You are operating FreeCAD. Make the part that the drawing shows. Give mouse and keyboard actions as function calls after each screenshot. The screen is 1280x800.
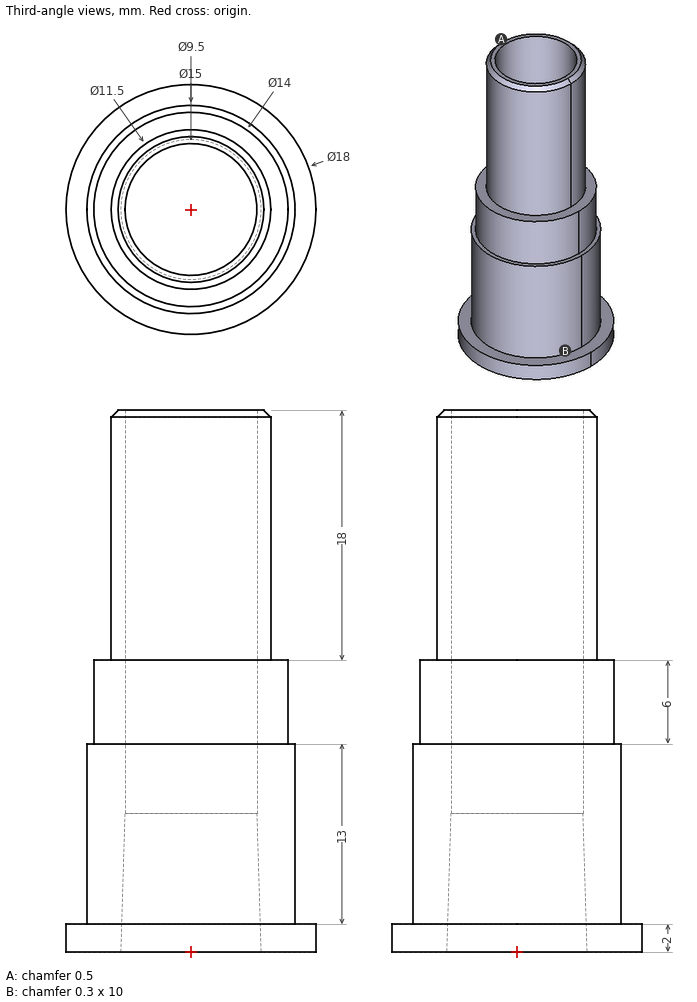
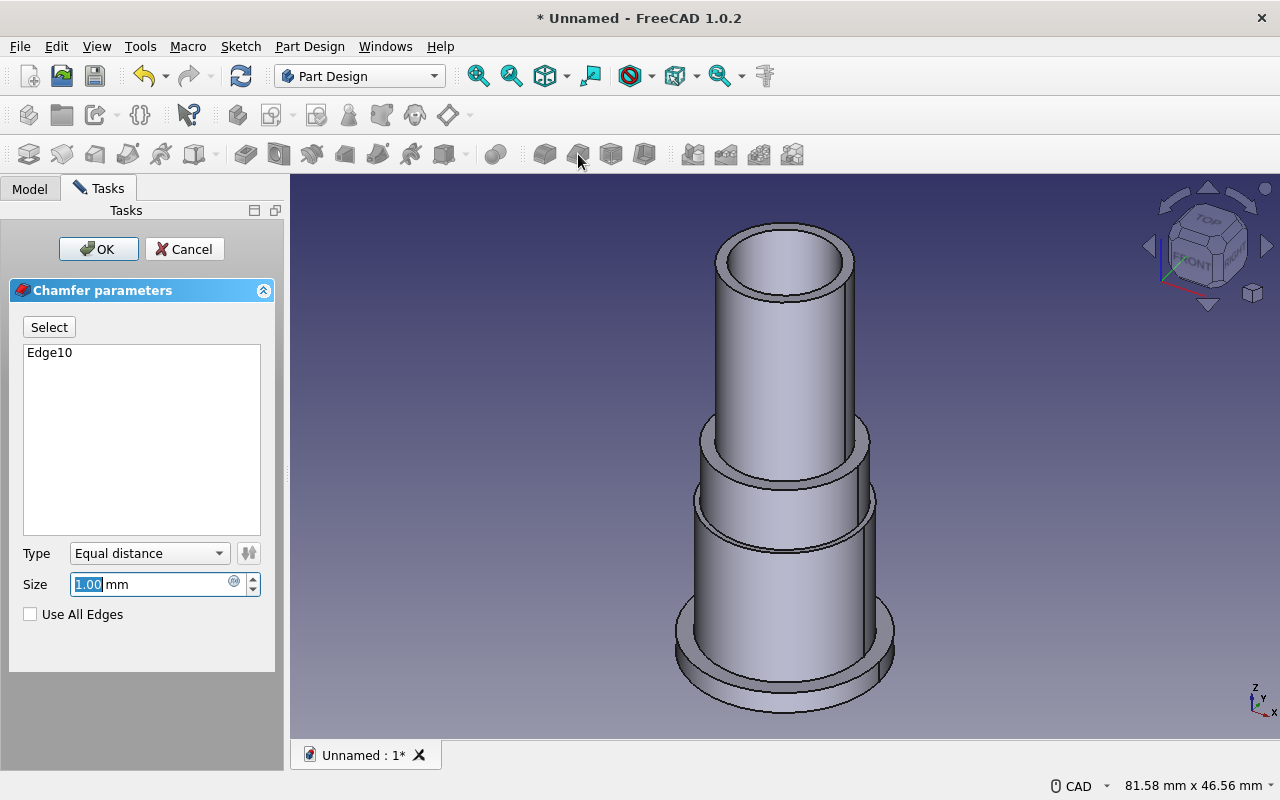
text(0.5)
key(Tab)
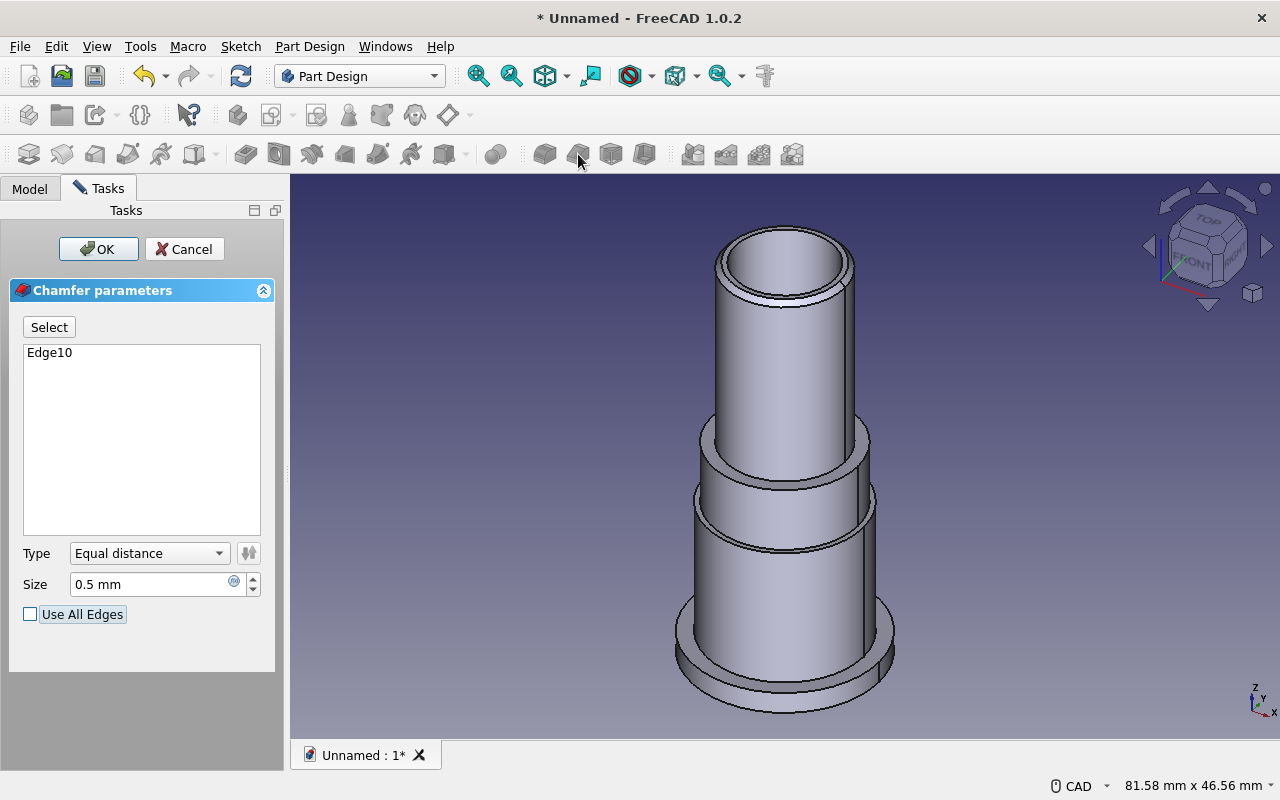
click(99, 249)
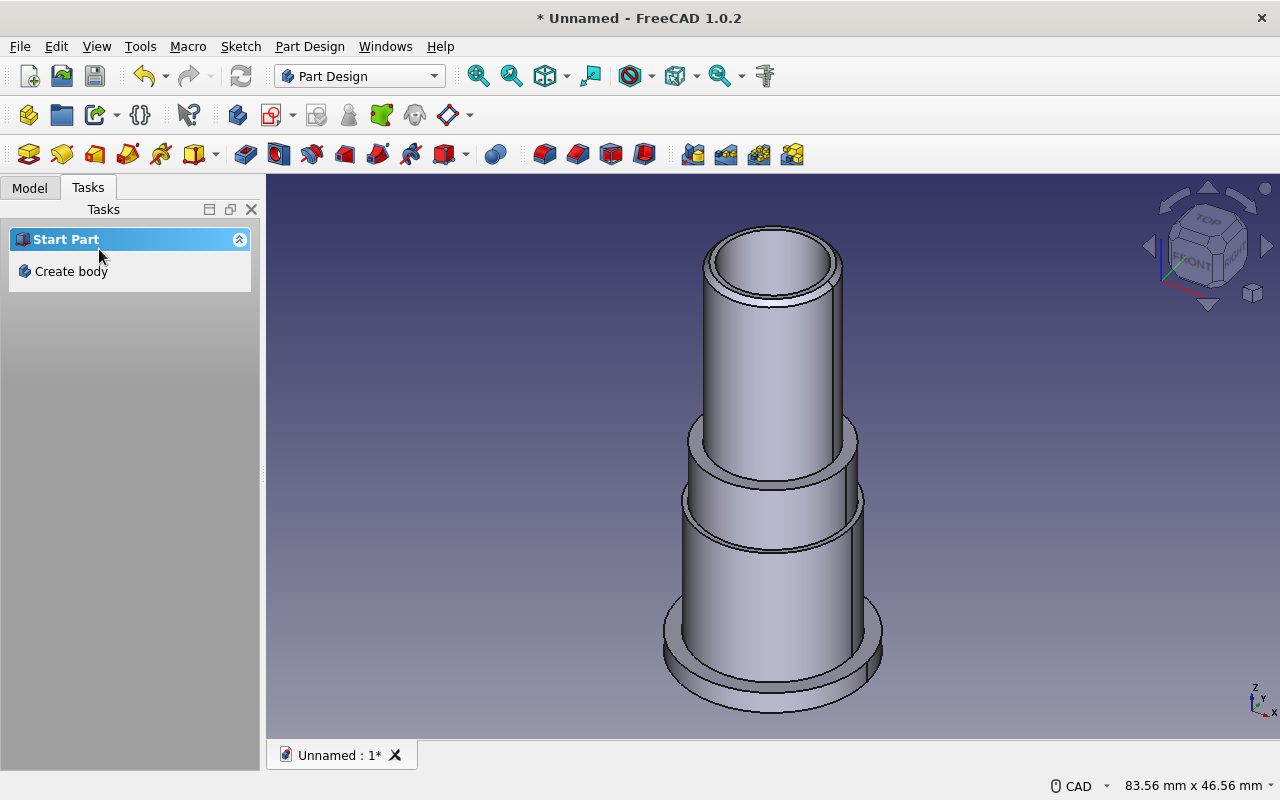
key(0)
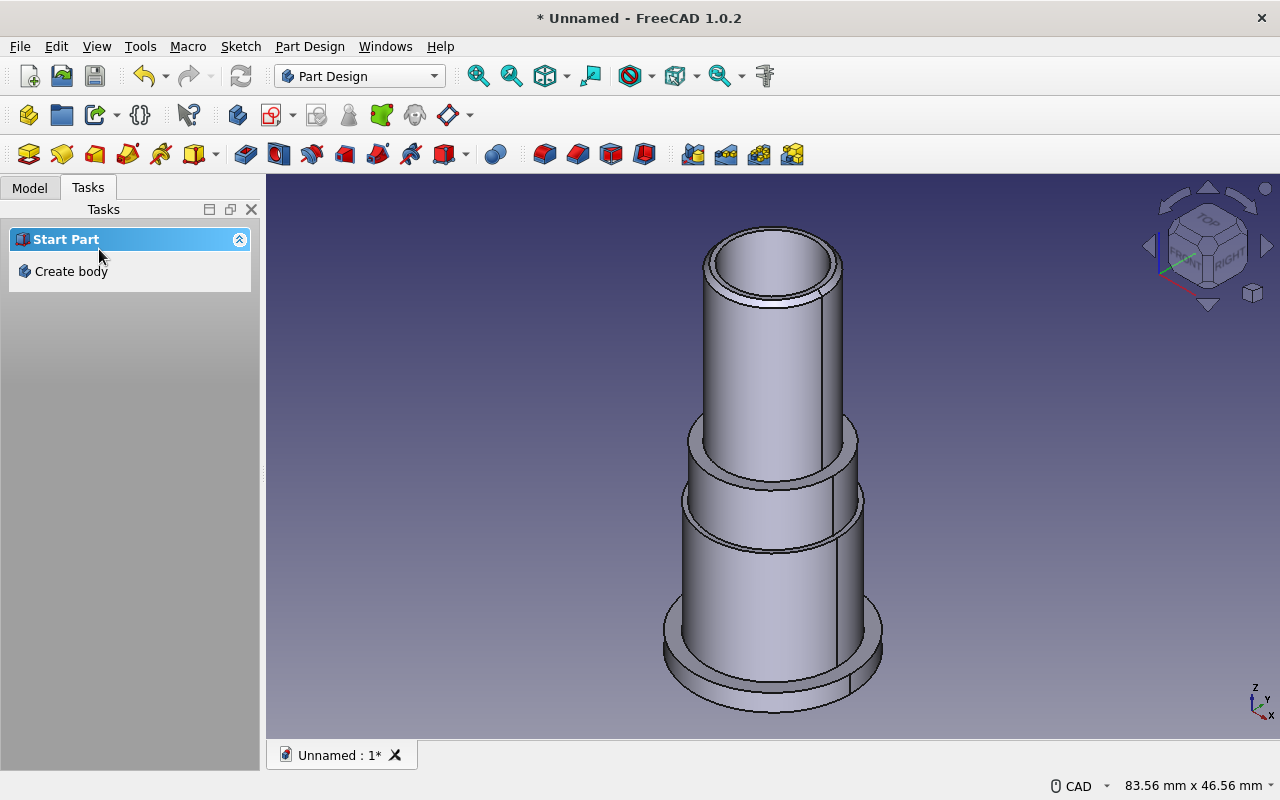
click(479, 76)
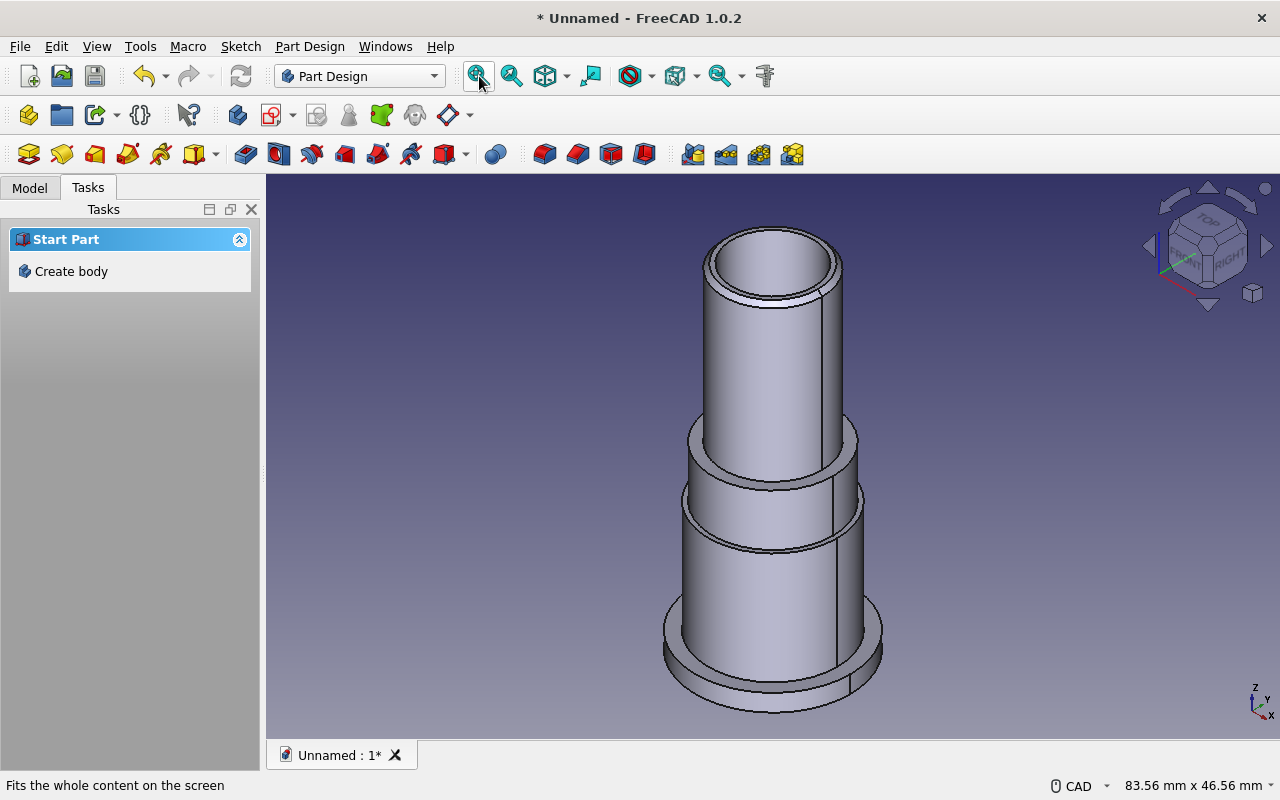
key(2)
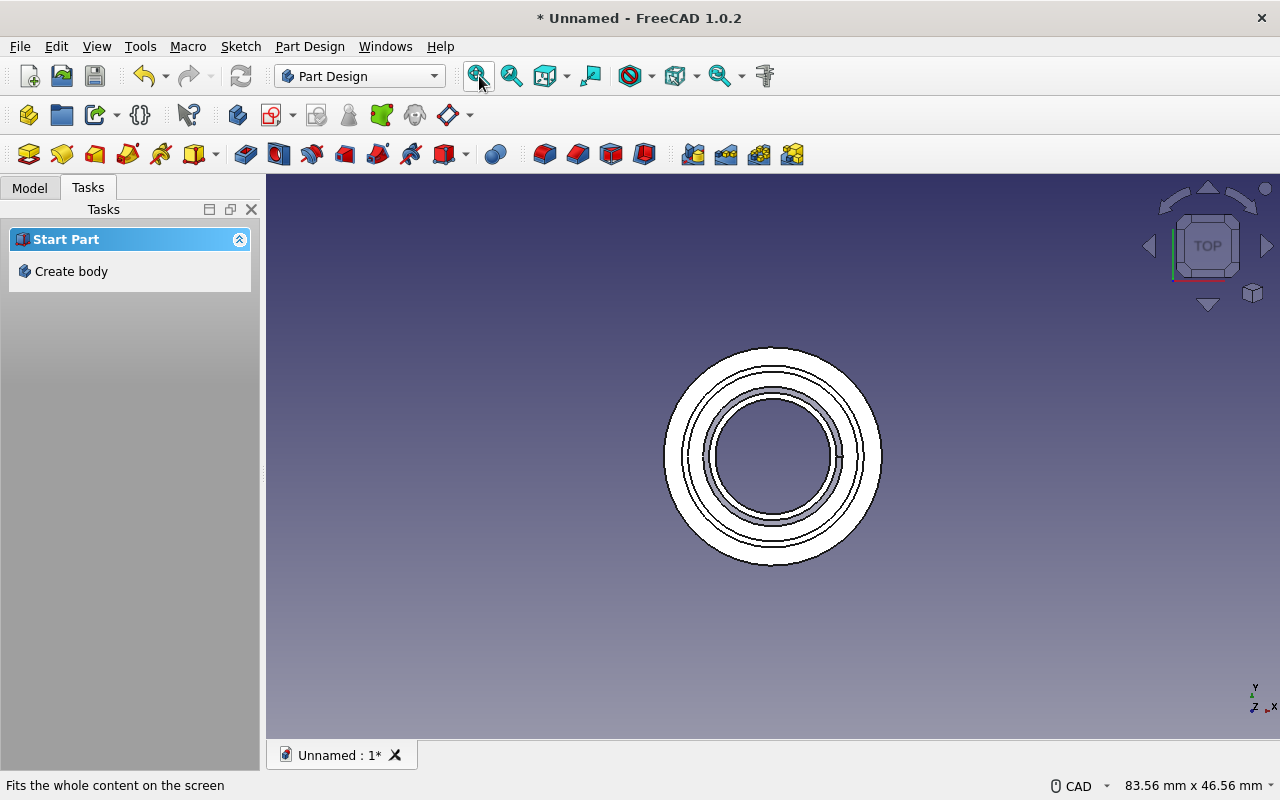
click(479, 76)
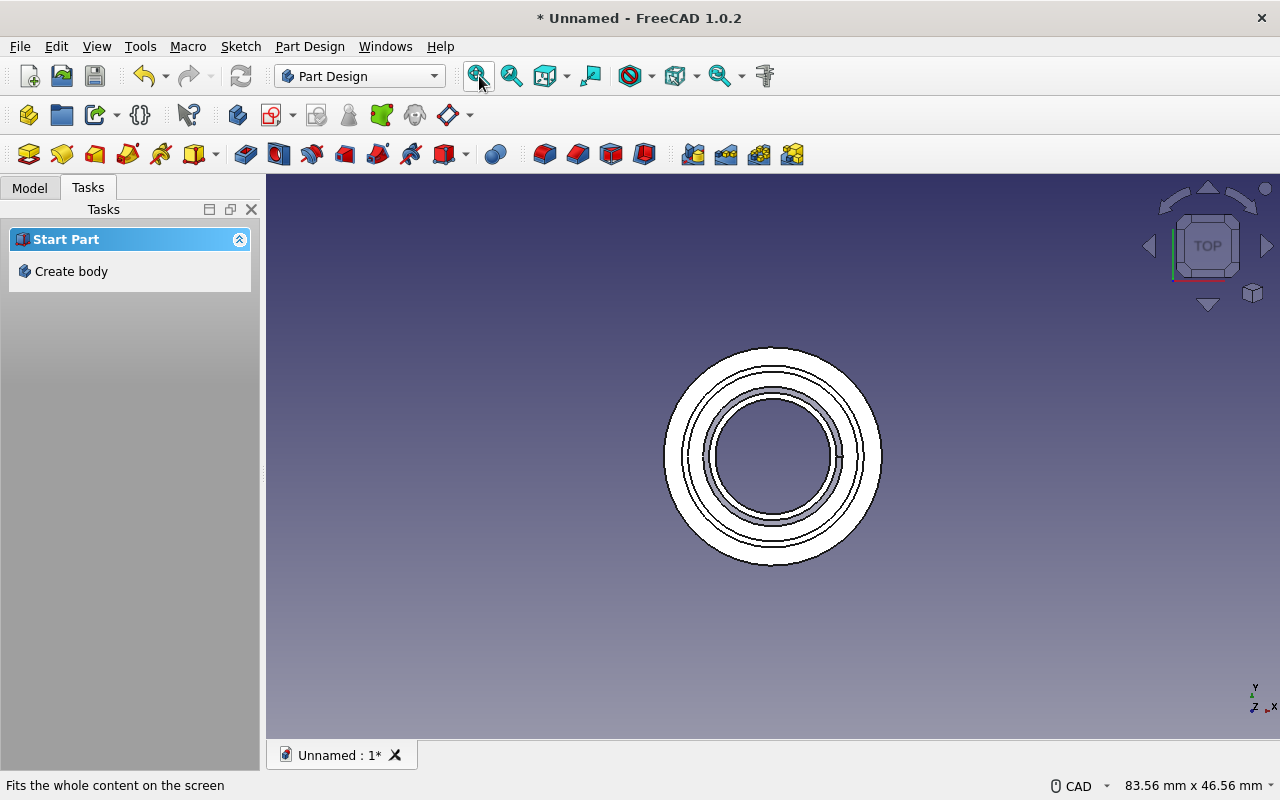
key(1)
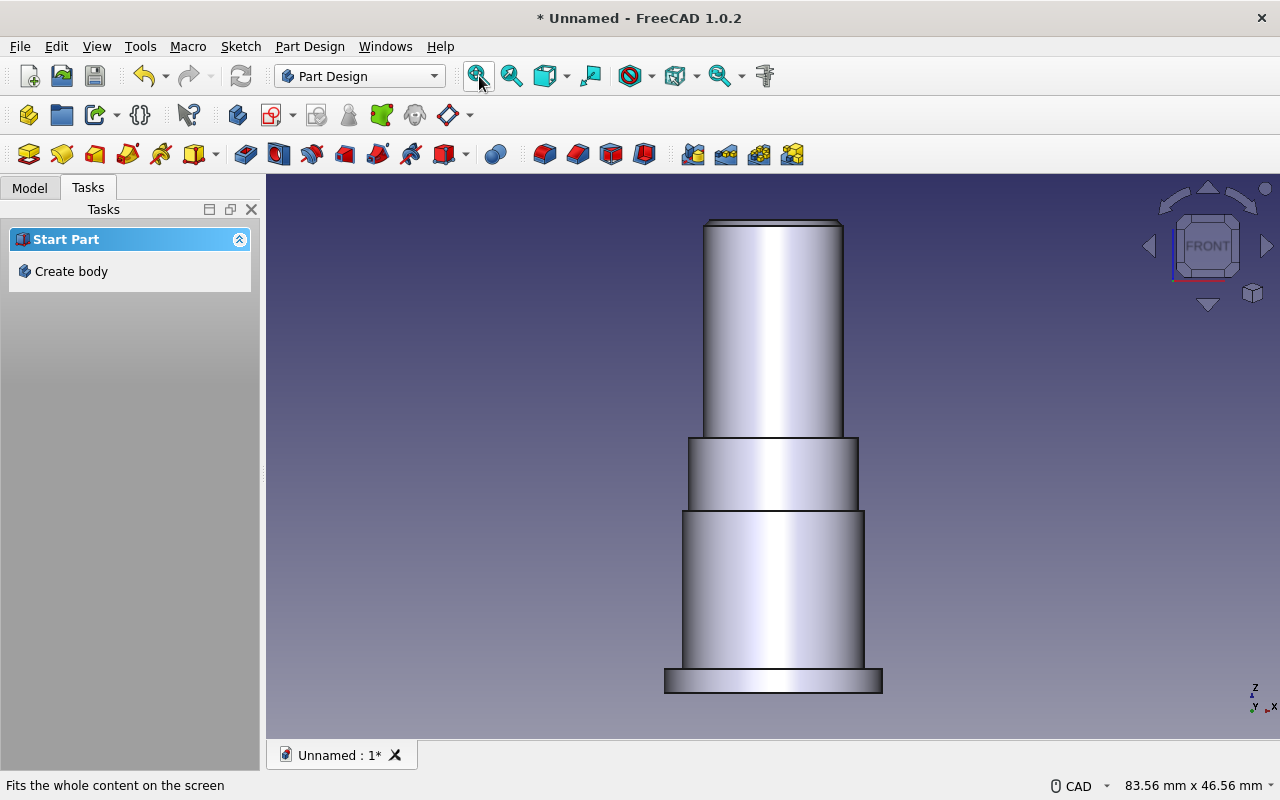
key(3)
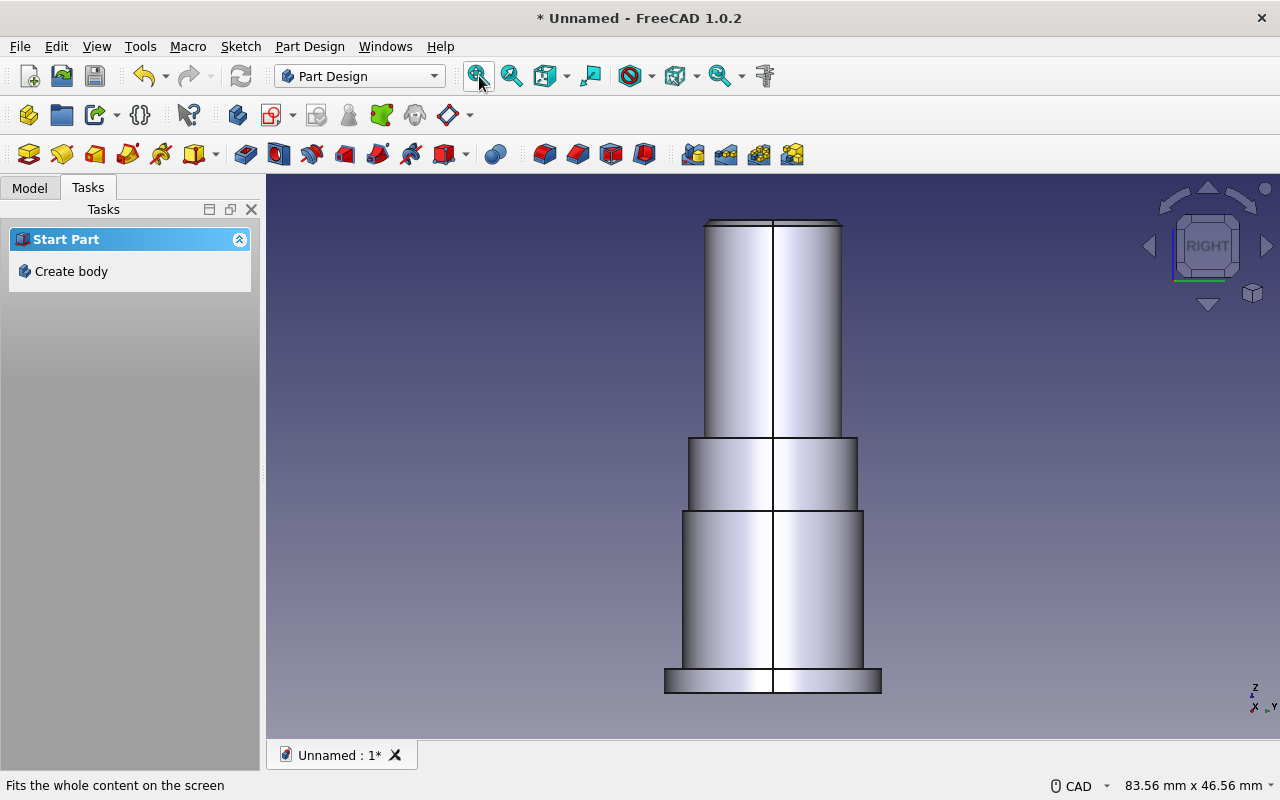
key(5)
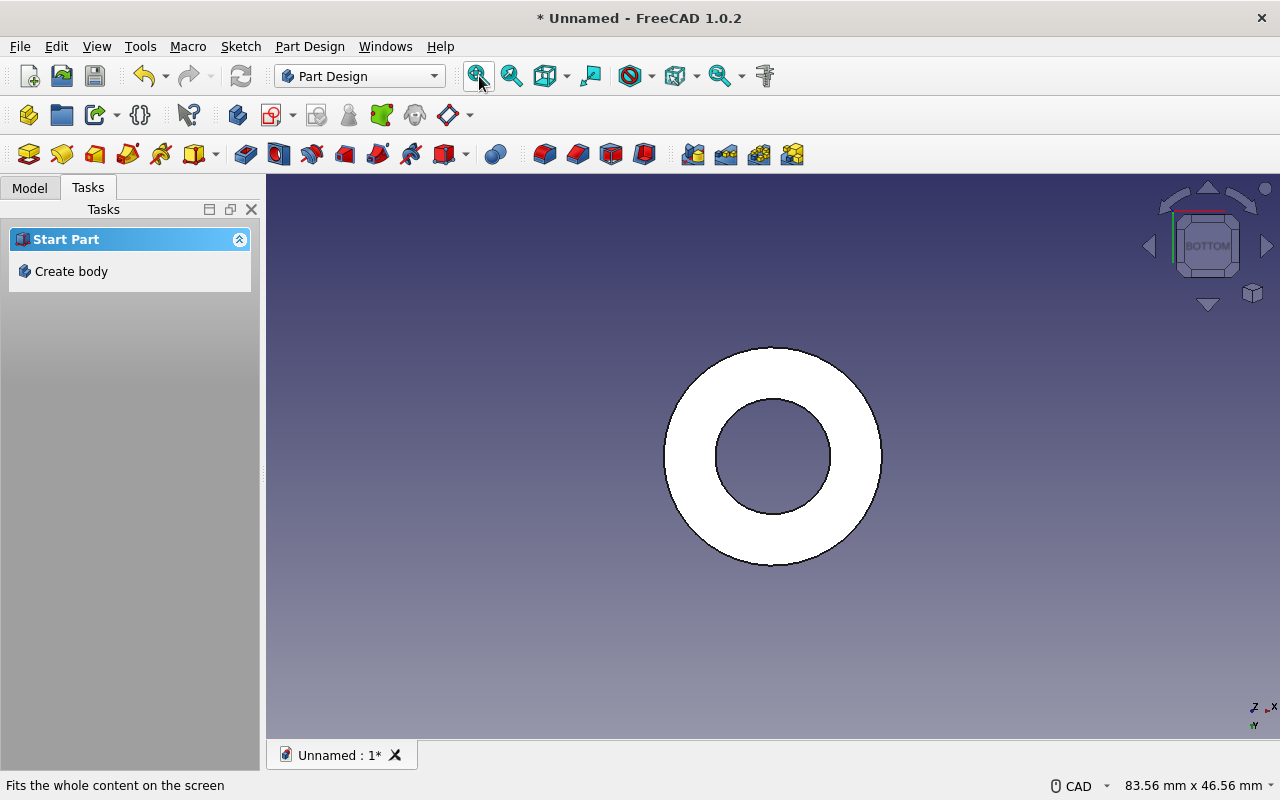
click(479, 76)